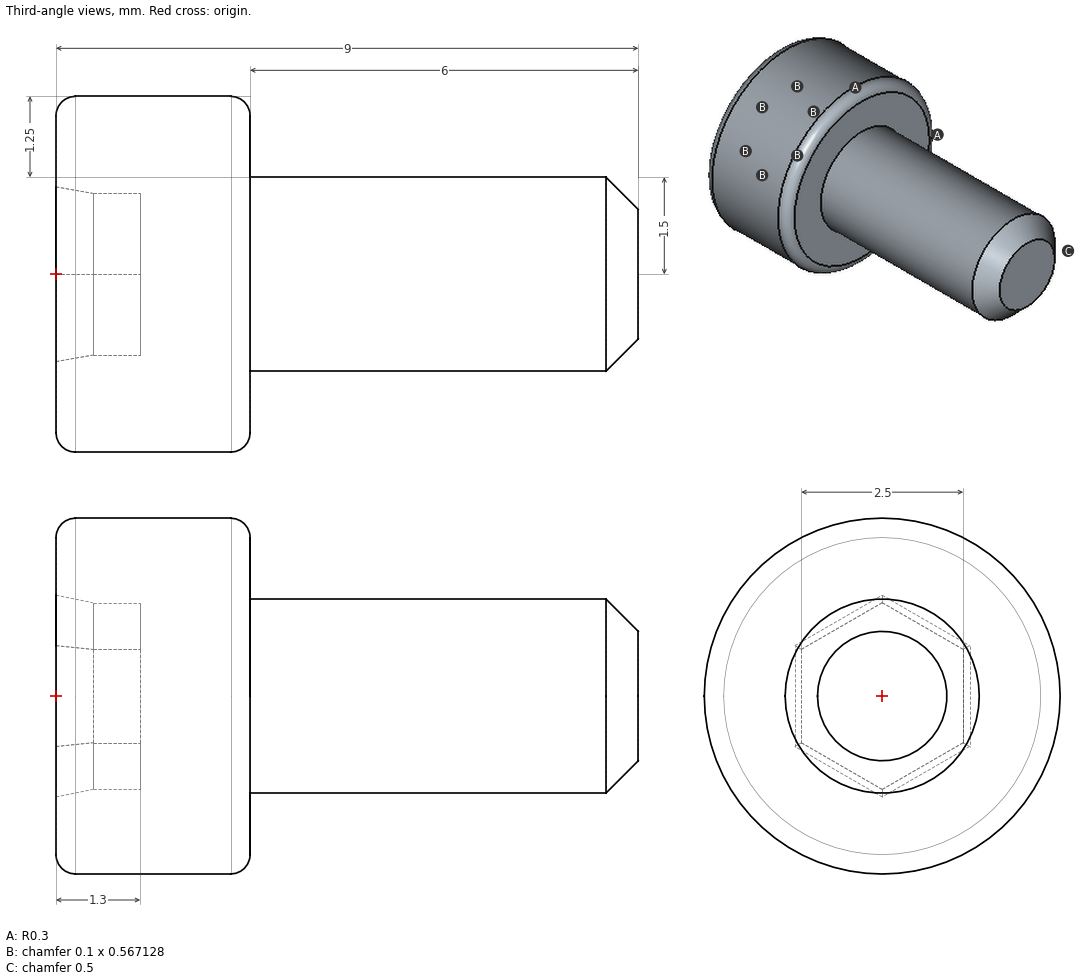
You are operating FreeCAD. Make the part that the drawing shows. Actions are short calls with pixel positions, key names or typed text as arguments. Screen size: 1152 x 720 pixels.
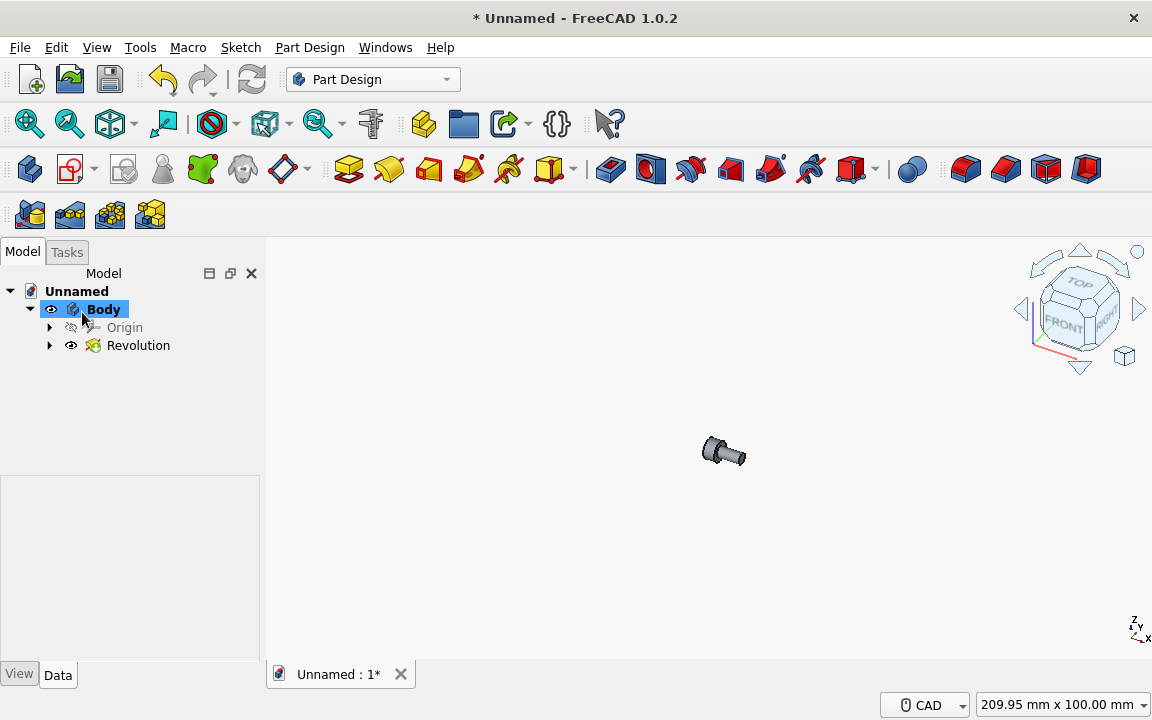
click(30, 124)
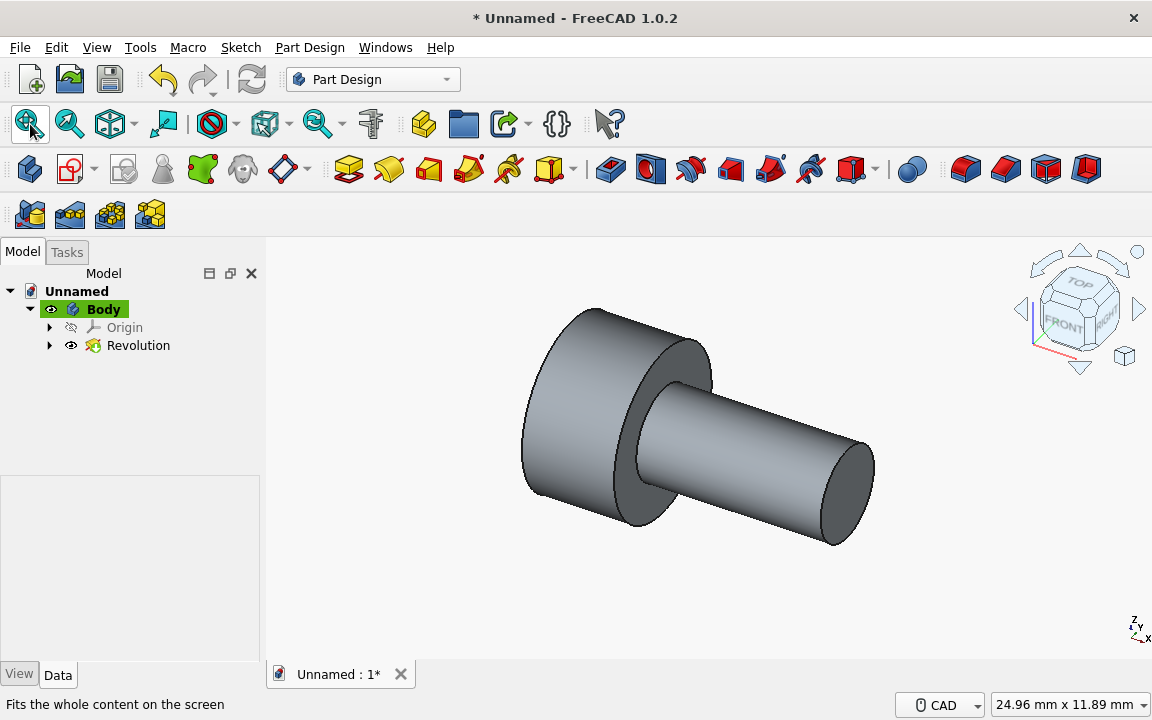
click(70, 170)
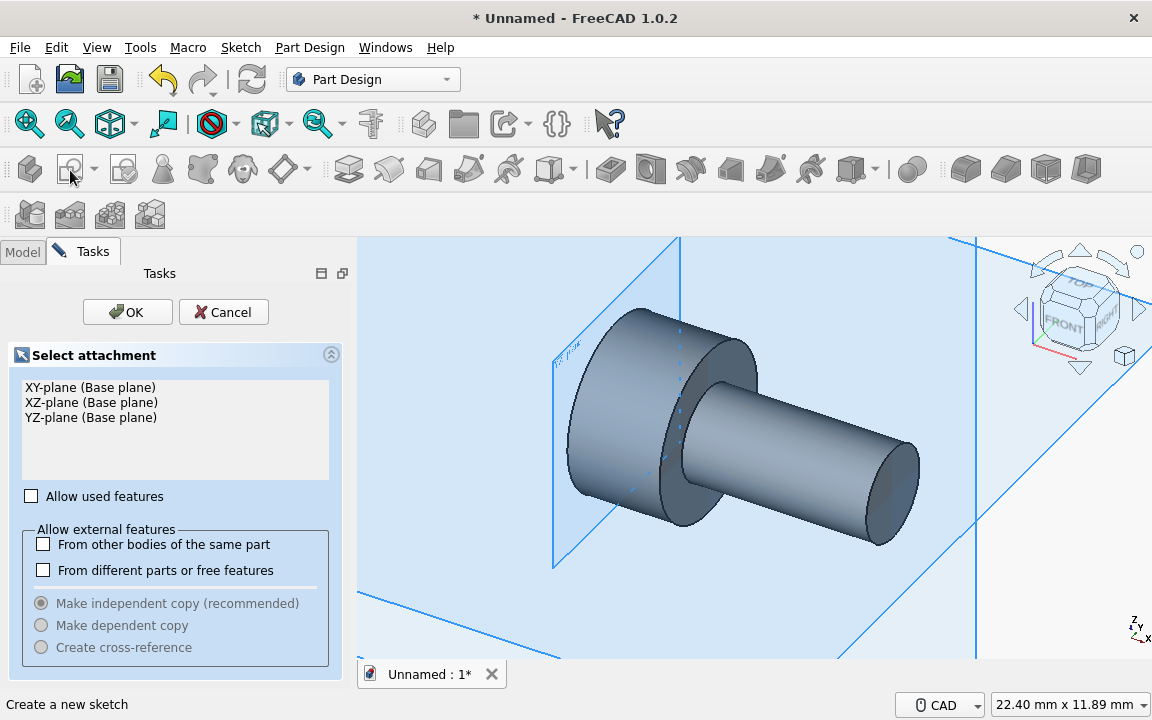
click(82, 418)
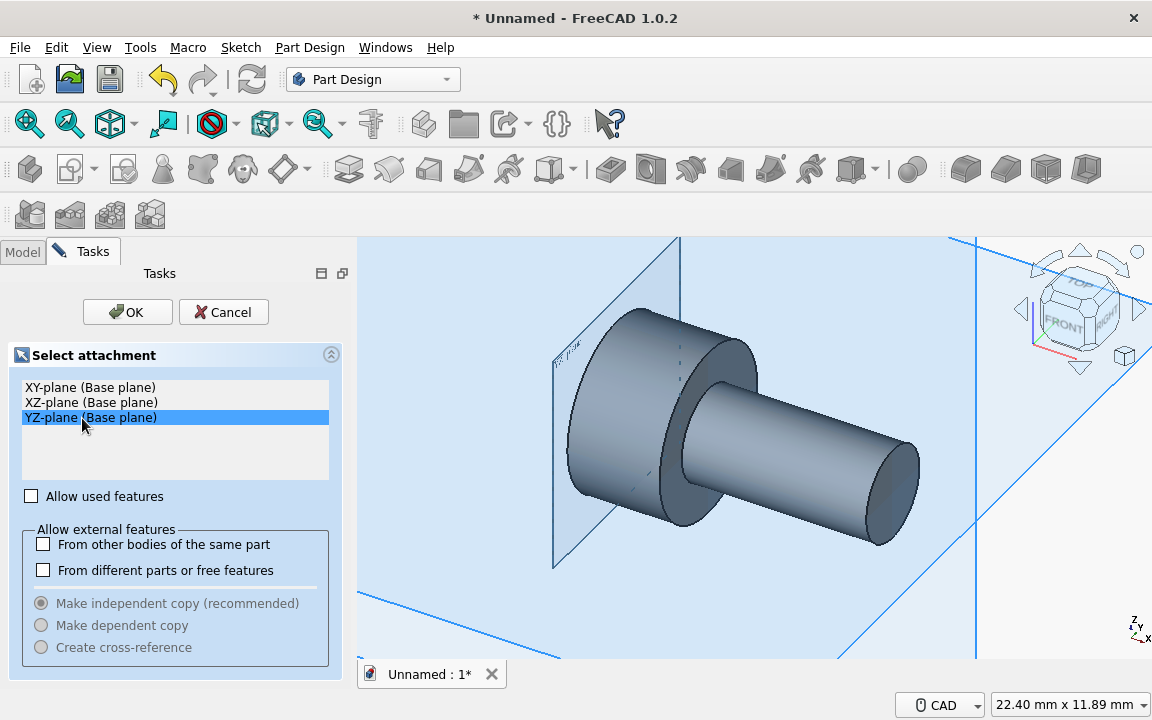
click(128, 312)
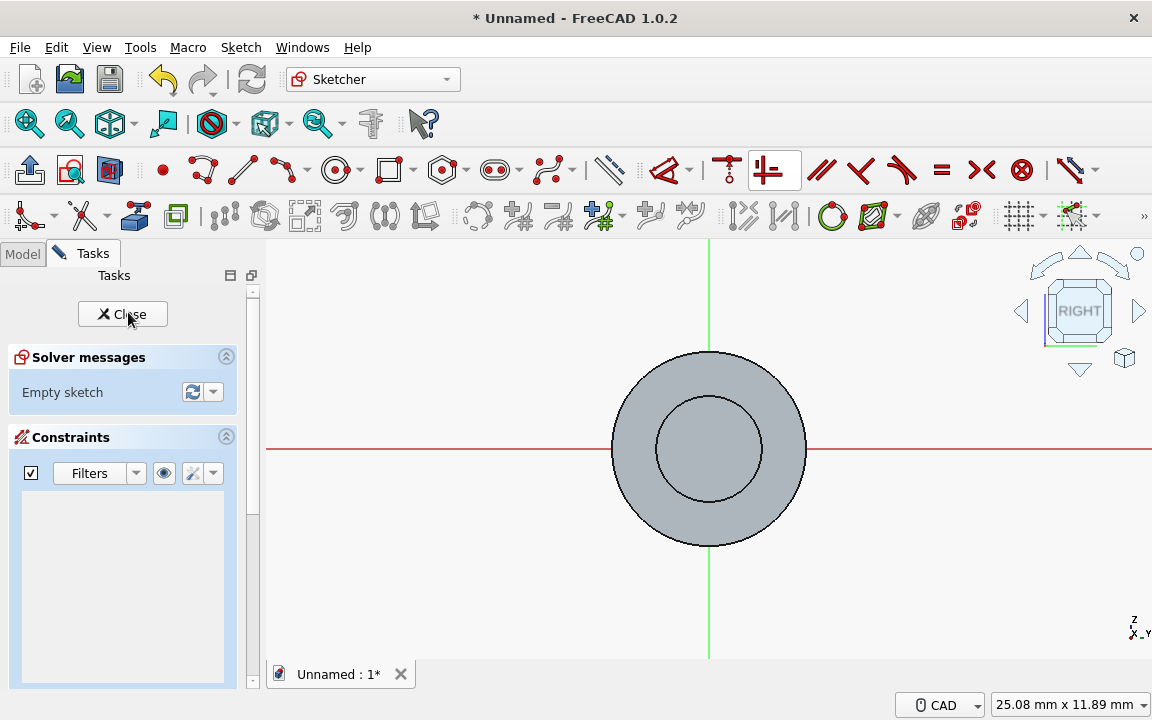
key(q)
key(s)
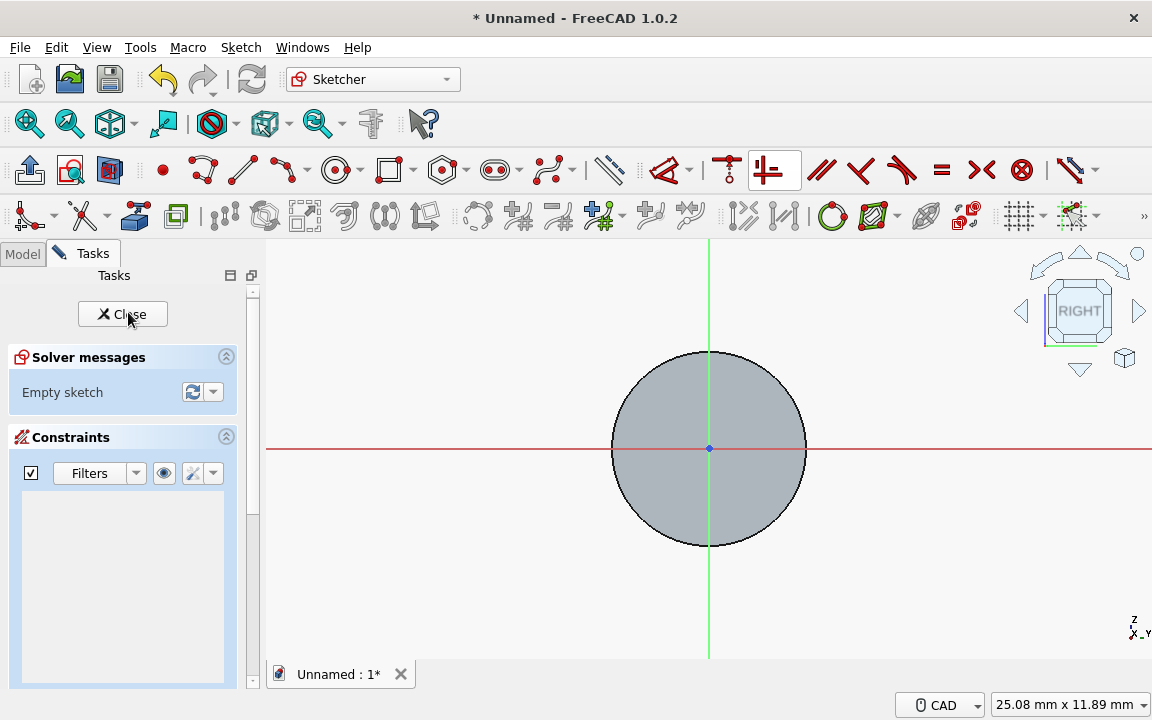
scroll(749, 449, up, 5)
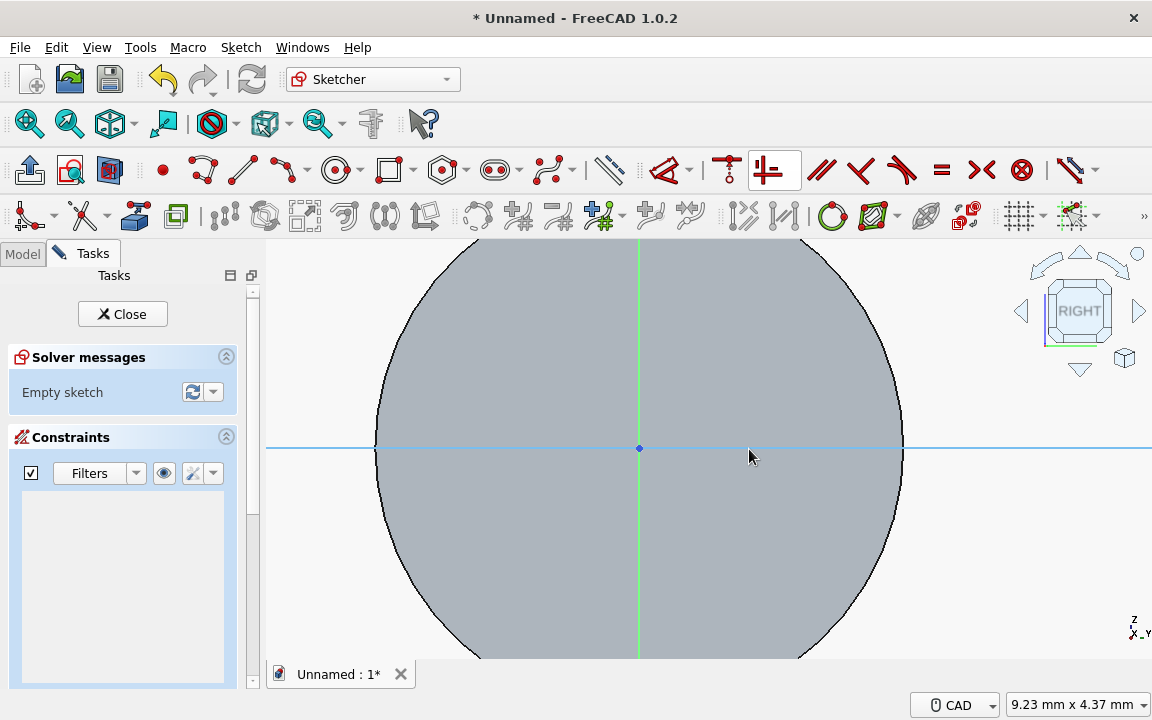
key(g)
key(p)
key(6)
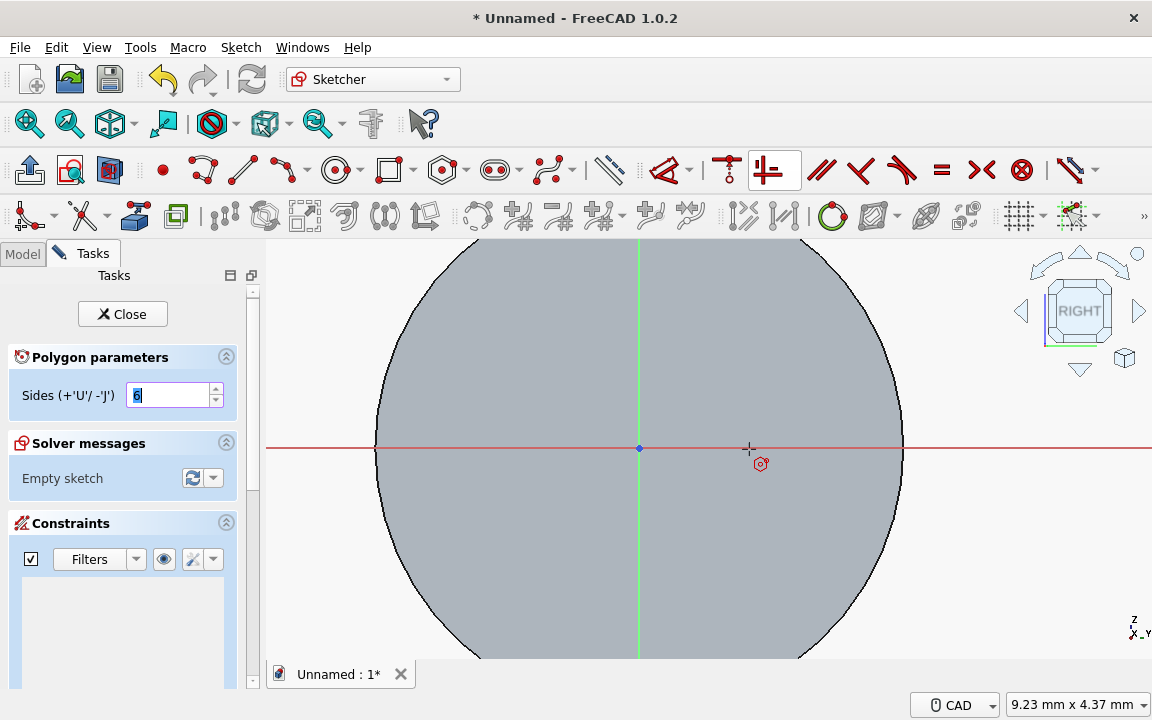
click(639, 448)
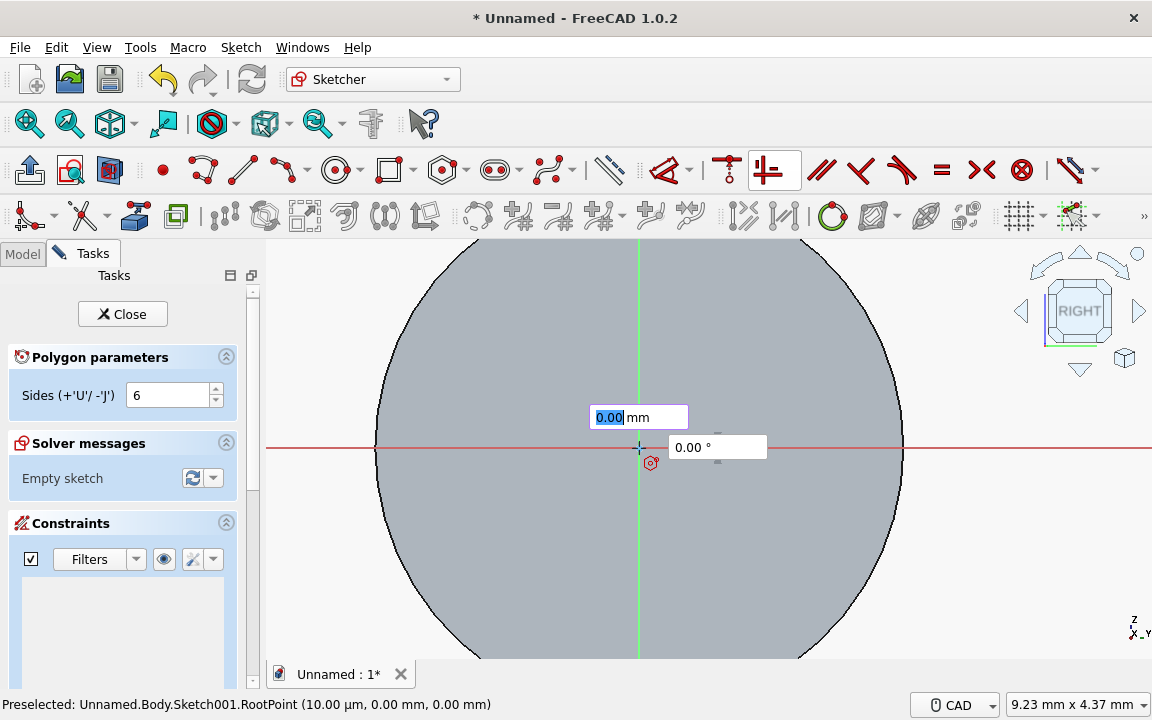
click(639, 587)
right_click(639, 587)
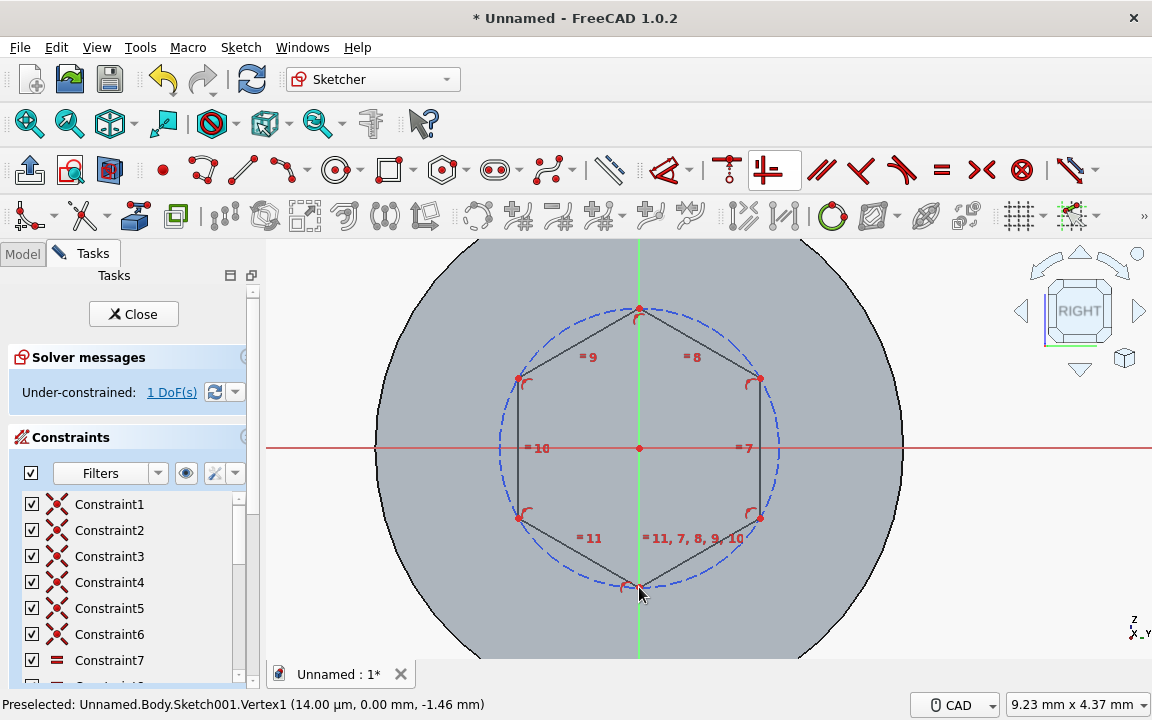
key(d)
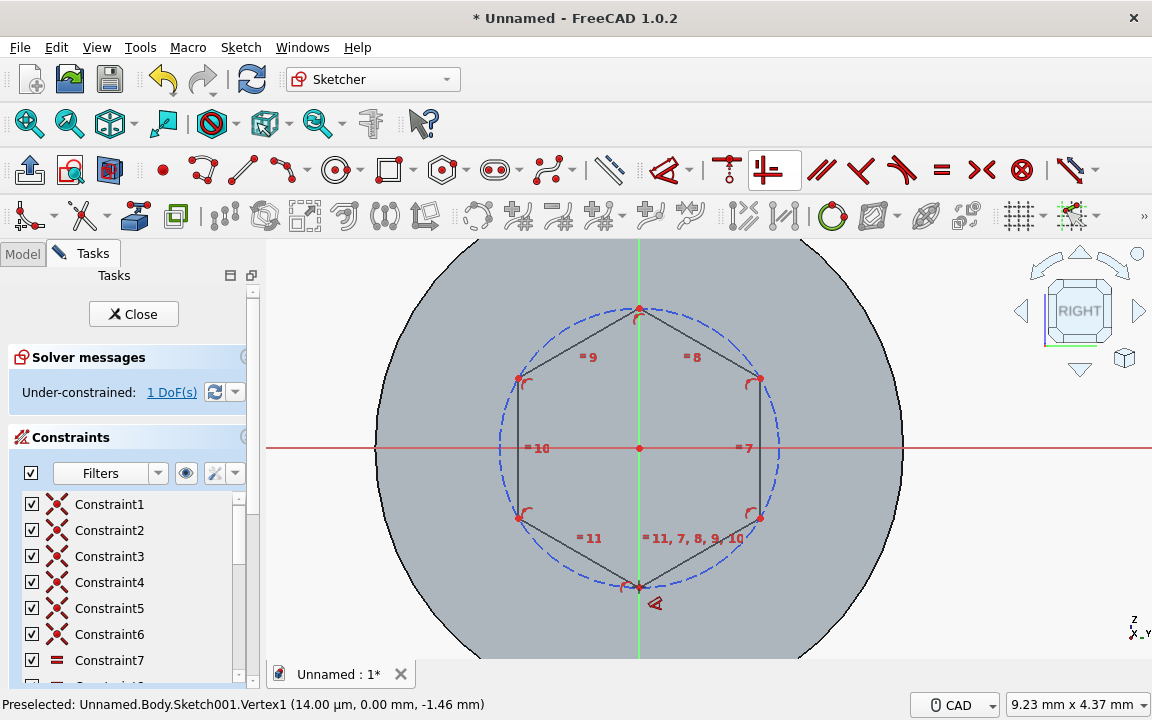
click(518, 378)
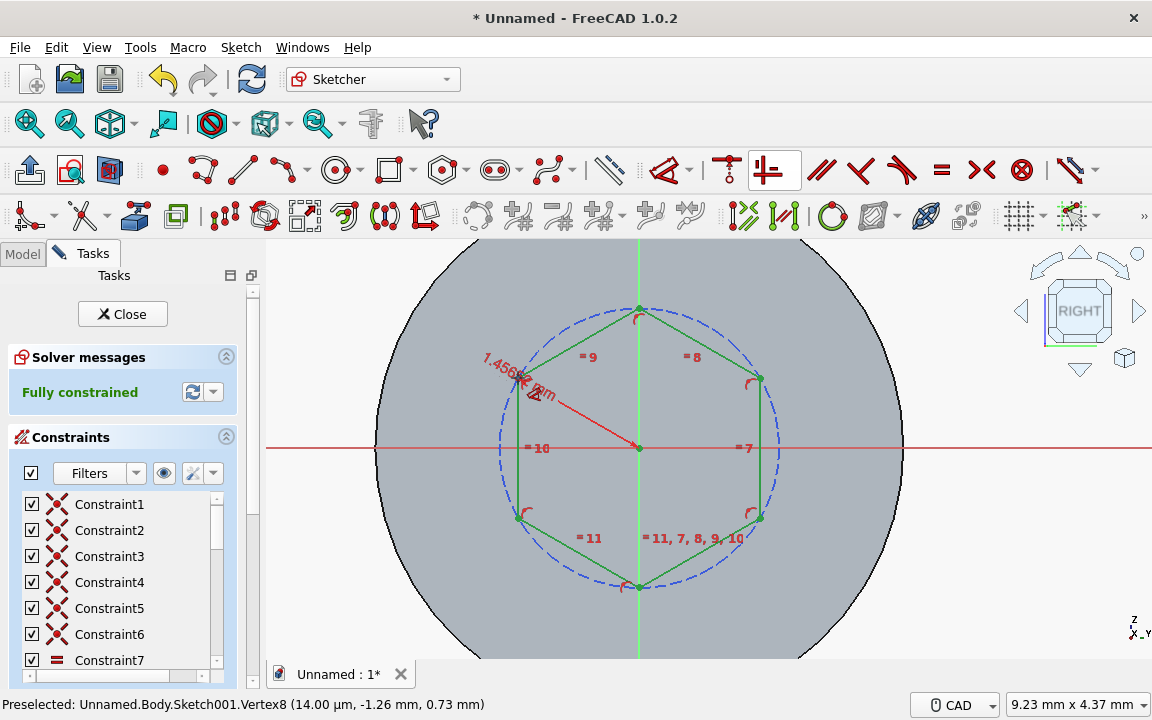
click(760, 518)
click(555, 320)